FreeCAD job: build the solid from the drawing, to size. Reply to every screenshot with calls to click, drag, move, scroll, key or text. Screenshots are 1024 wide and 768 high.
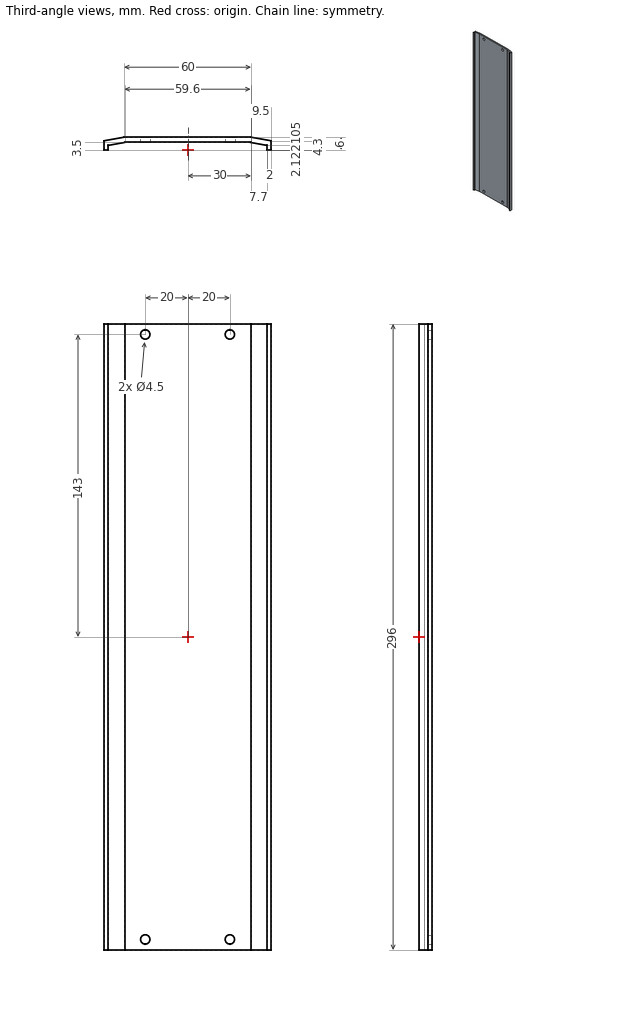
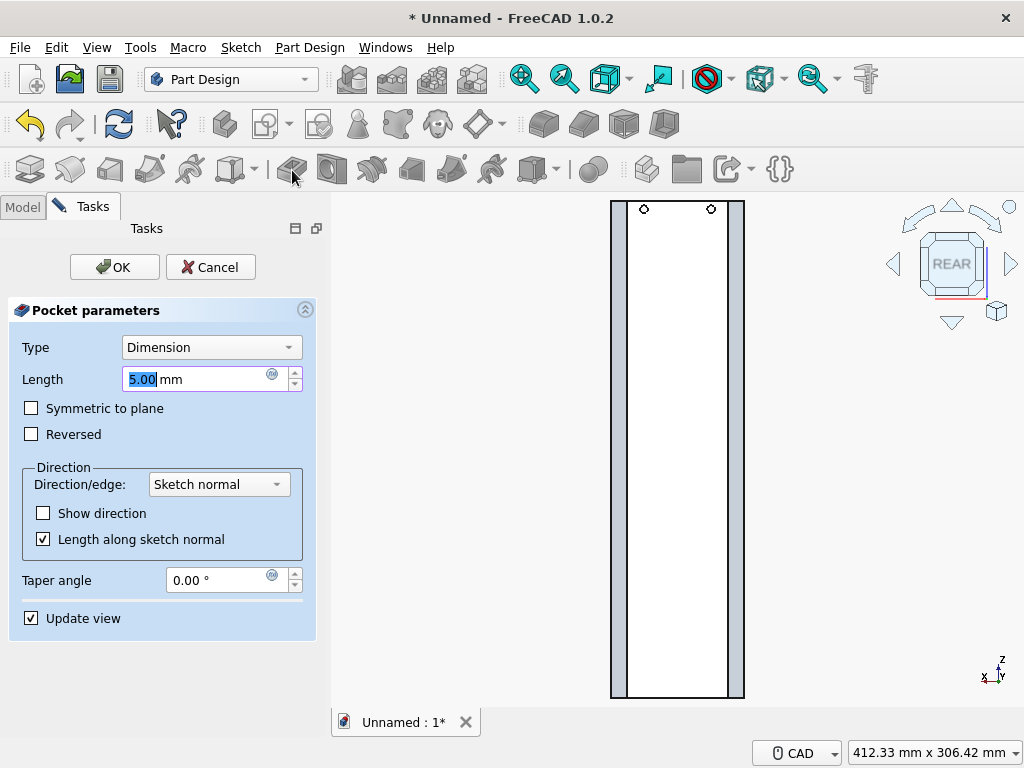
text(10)
key(Tab)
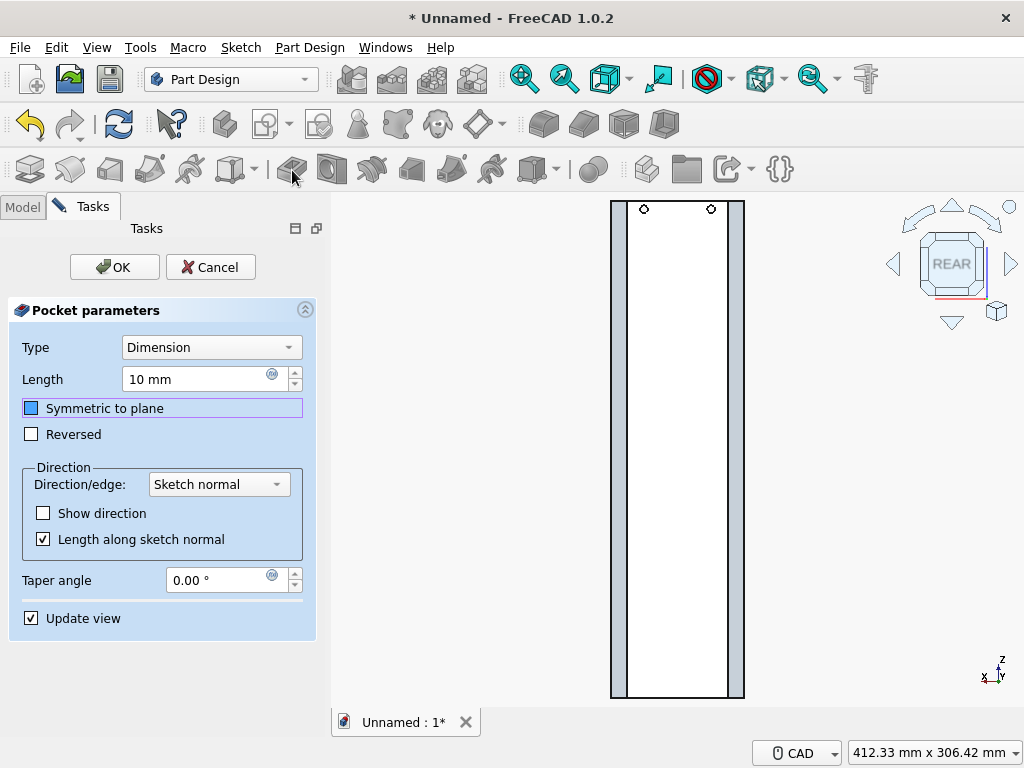
click(115, 267)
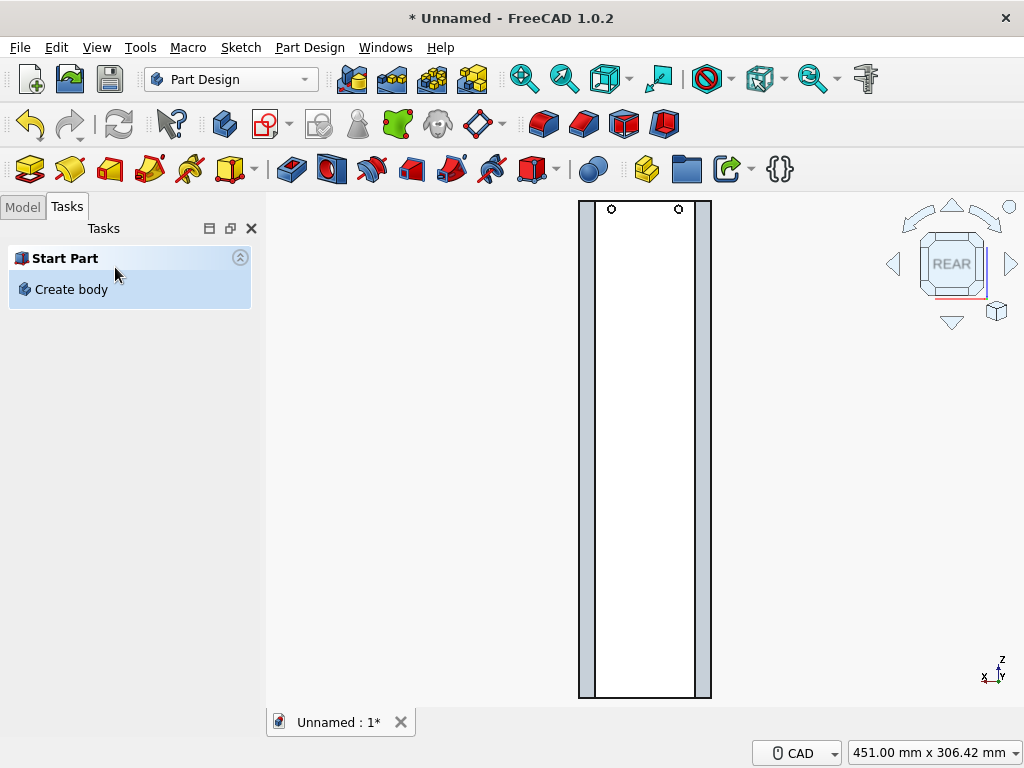
click(23, 206)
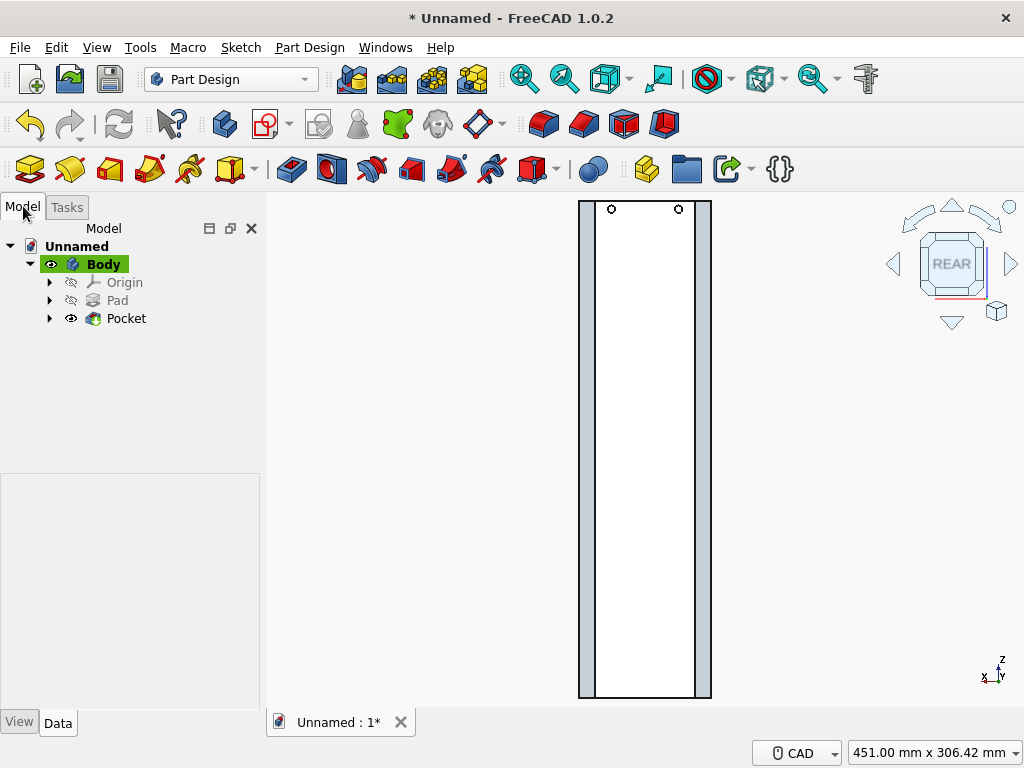
click(116, 318)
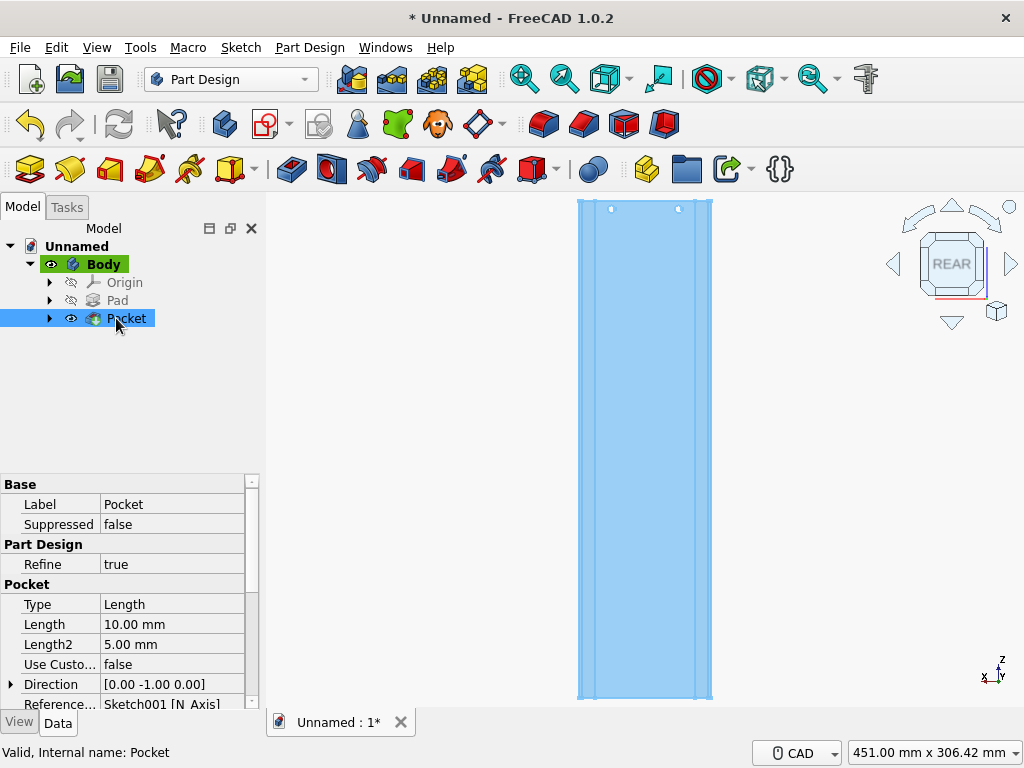
click(352, 80)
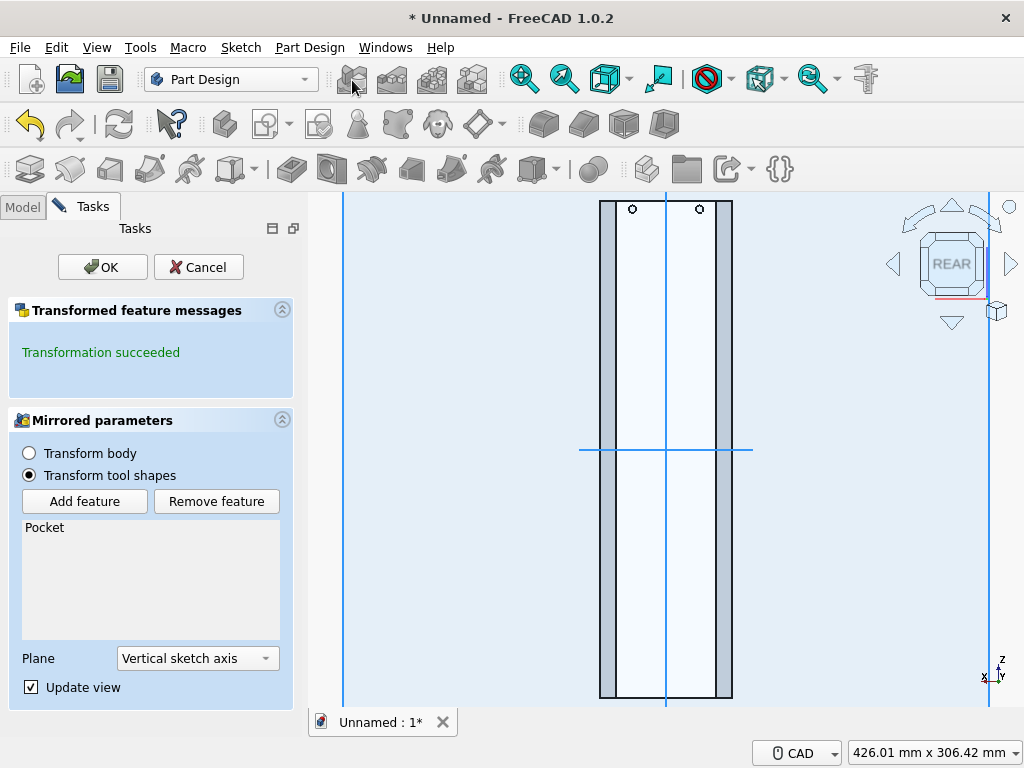
click(198, 658)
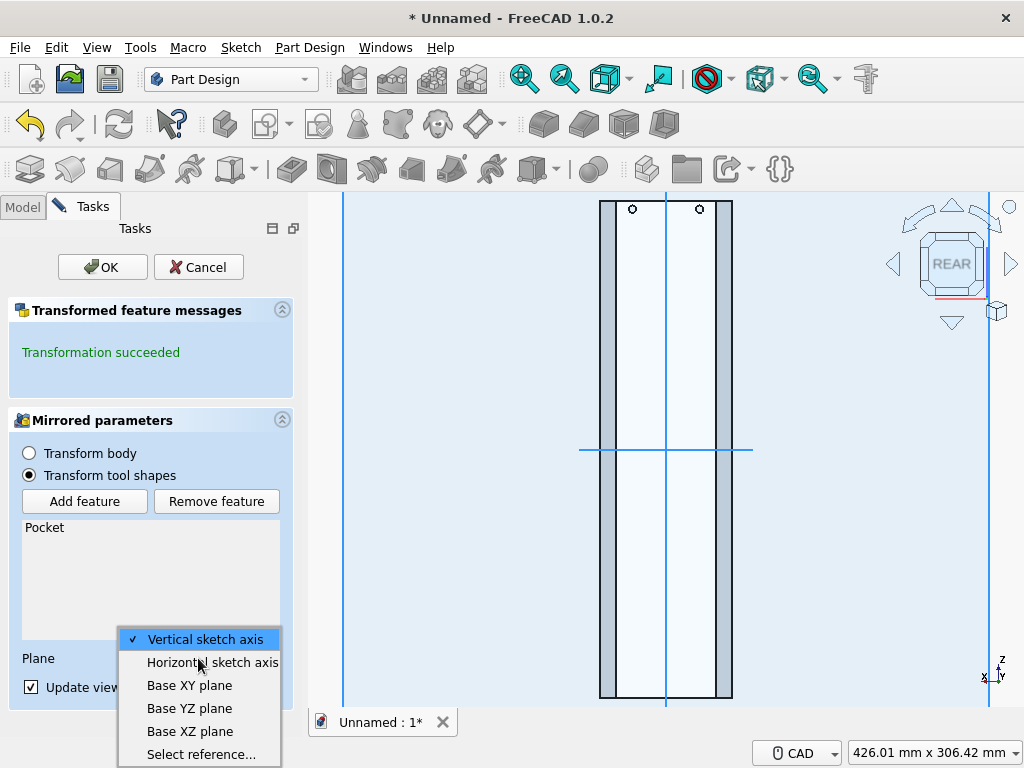
click(198, 686)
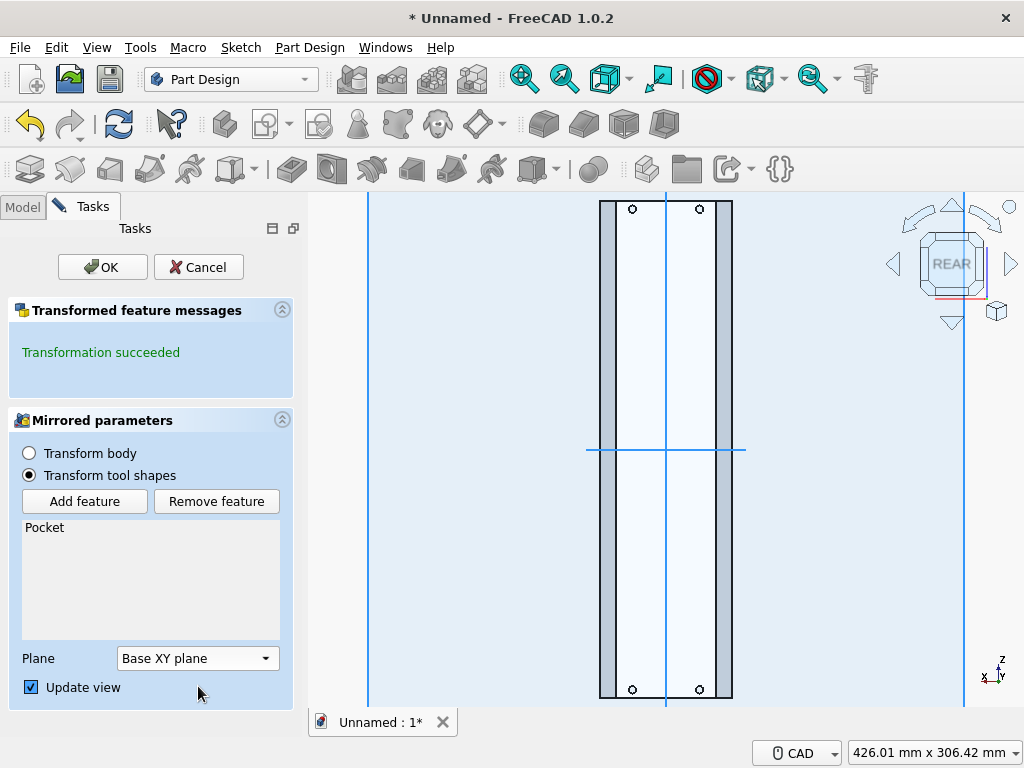
click(103, 267)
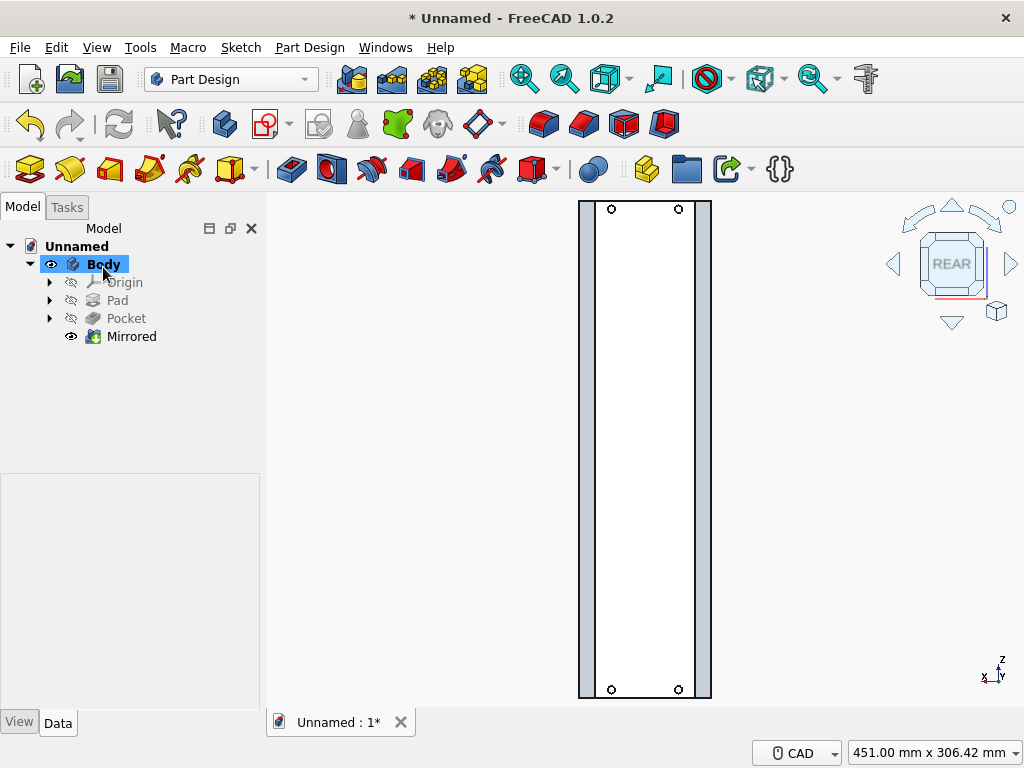
key(0)